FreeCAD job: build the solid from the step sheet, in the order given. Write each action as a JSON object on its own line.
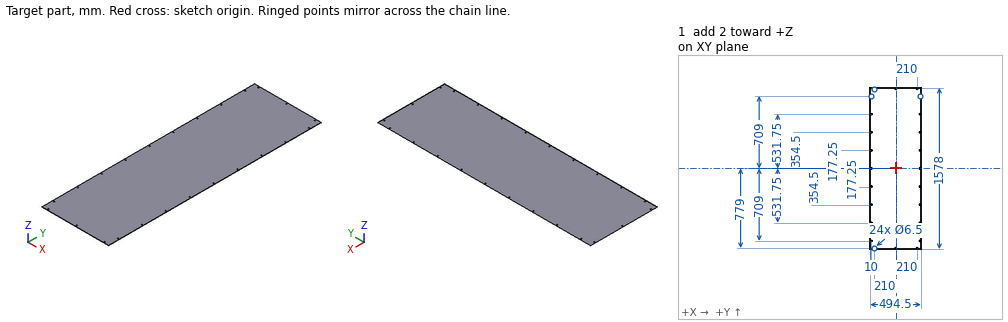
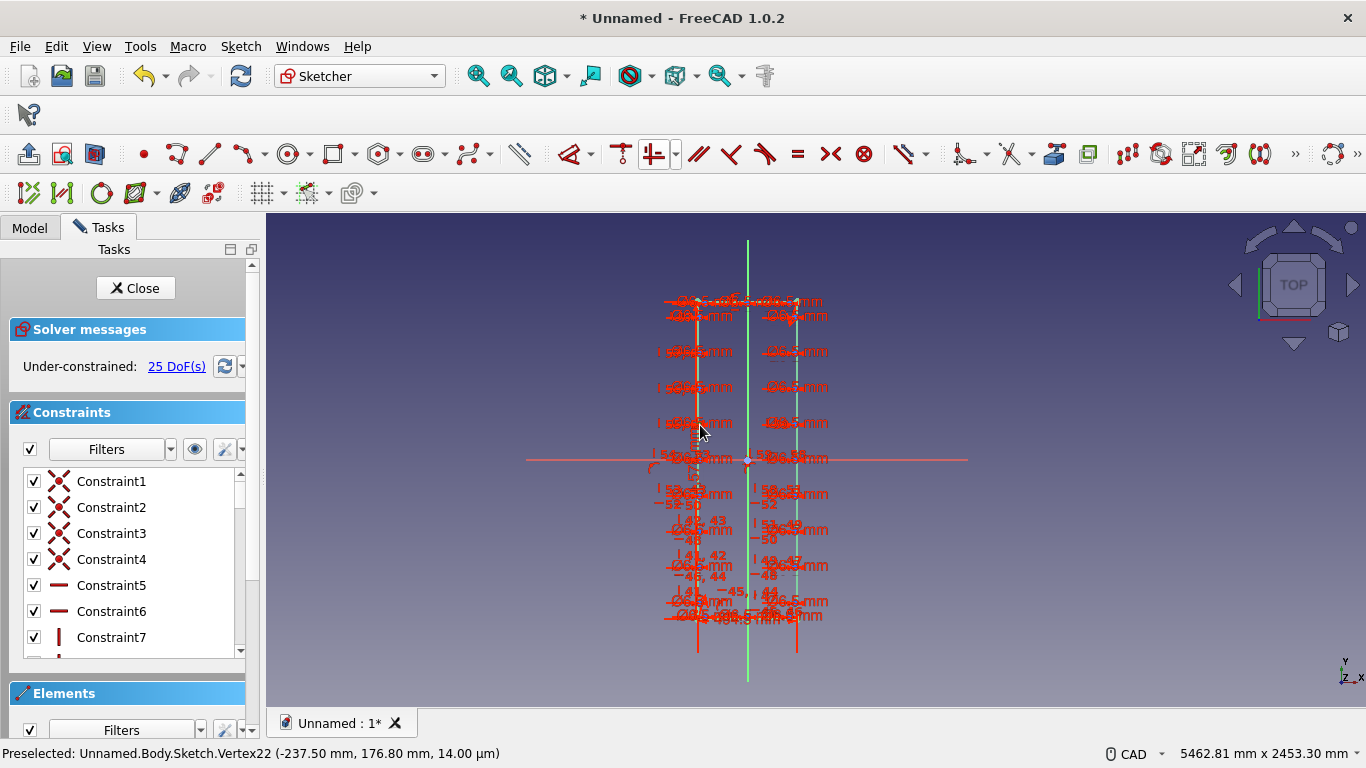
{"action": "left_click", "coordinate": [795, 425]}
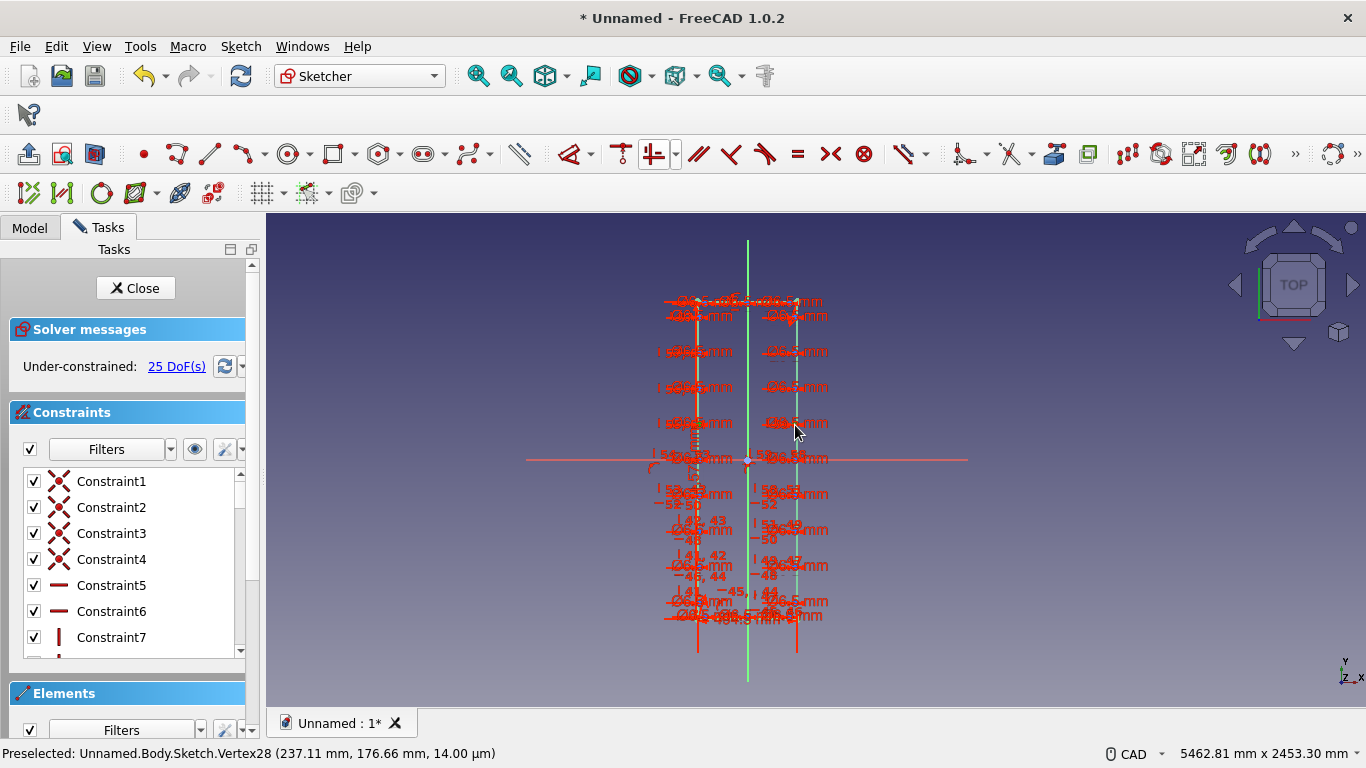
{"action": "left_click", "coordinate": [676, 154]}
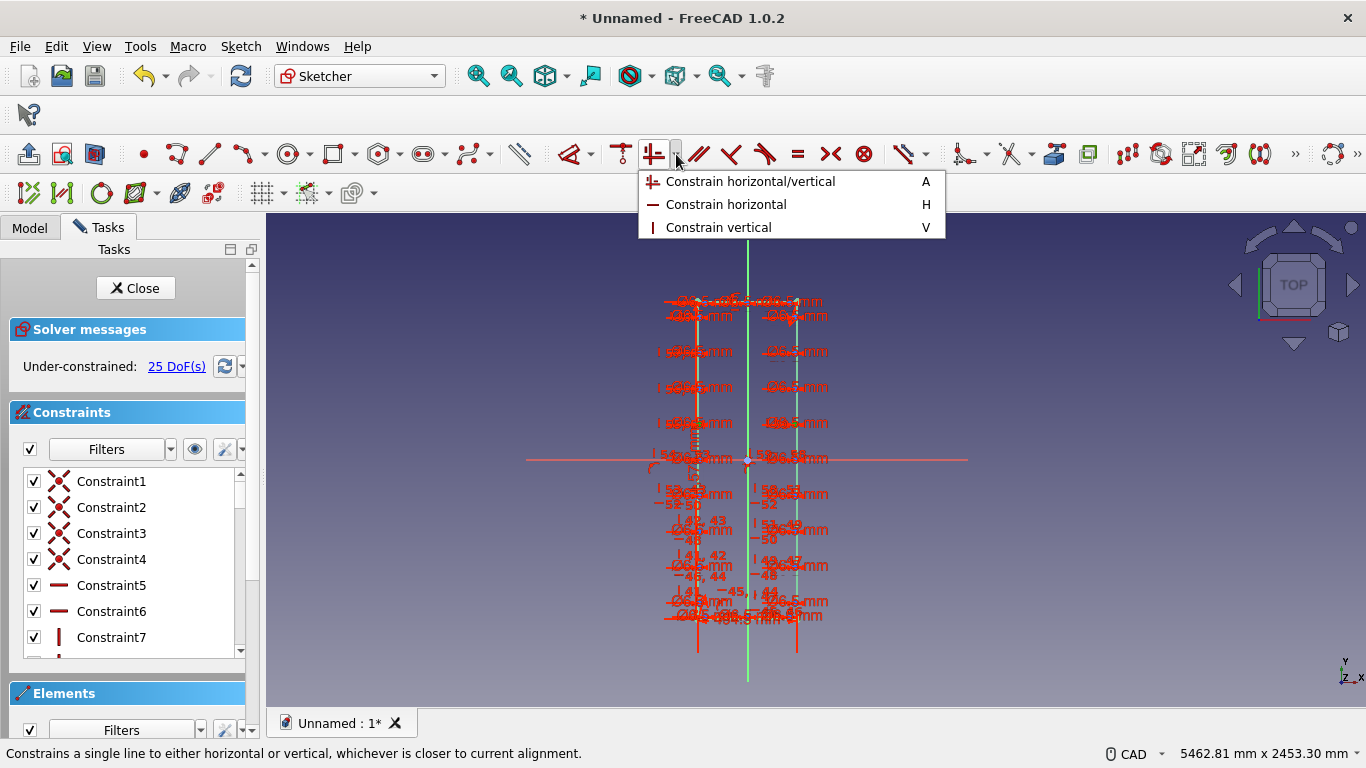
{"action": "left_click", "coordinate": [792, 204]}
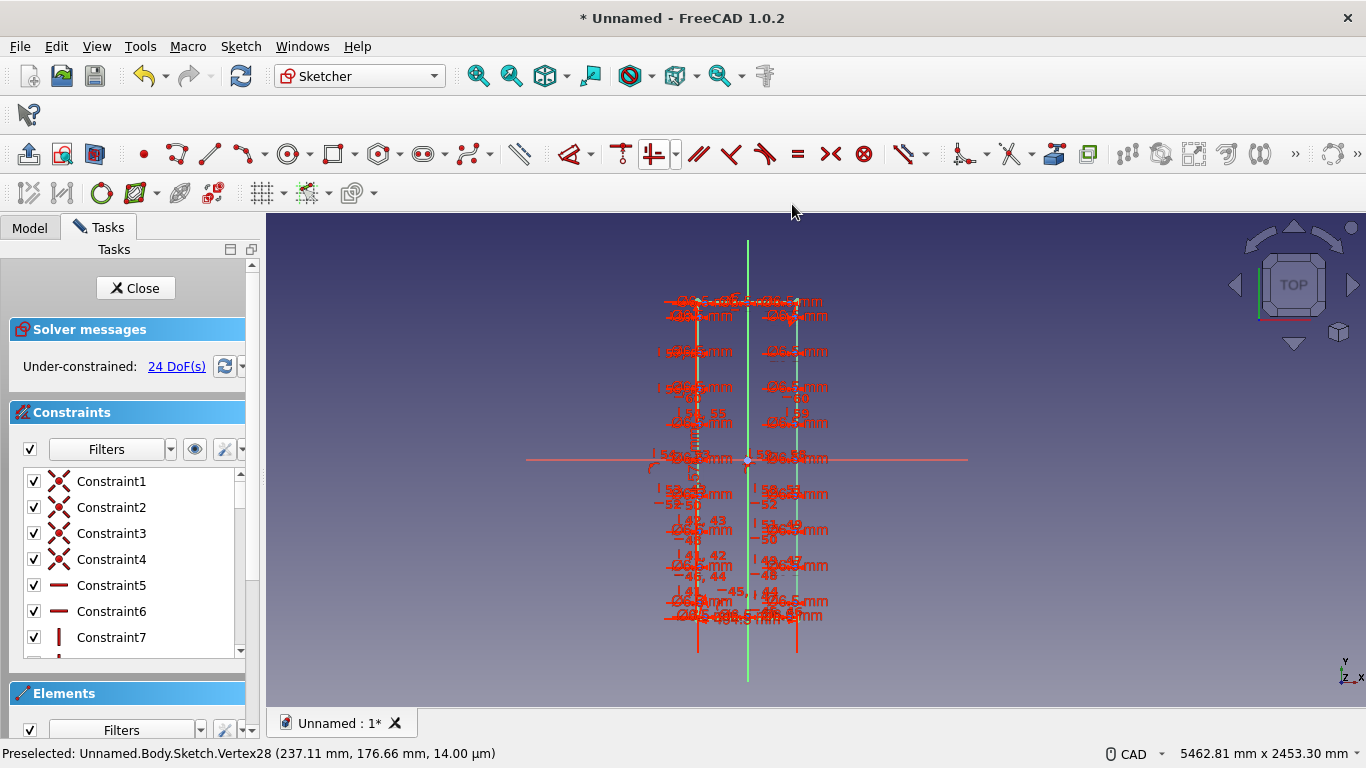
{"action": "left_click", "coordinate": [795, 425]}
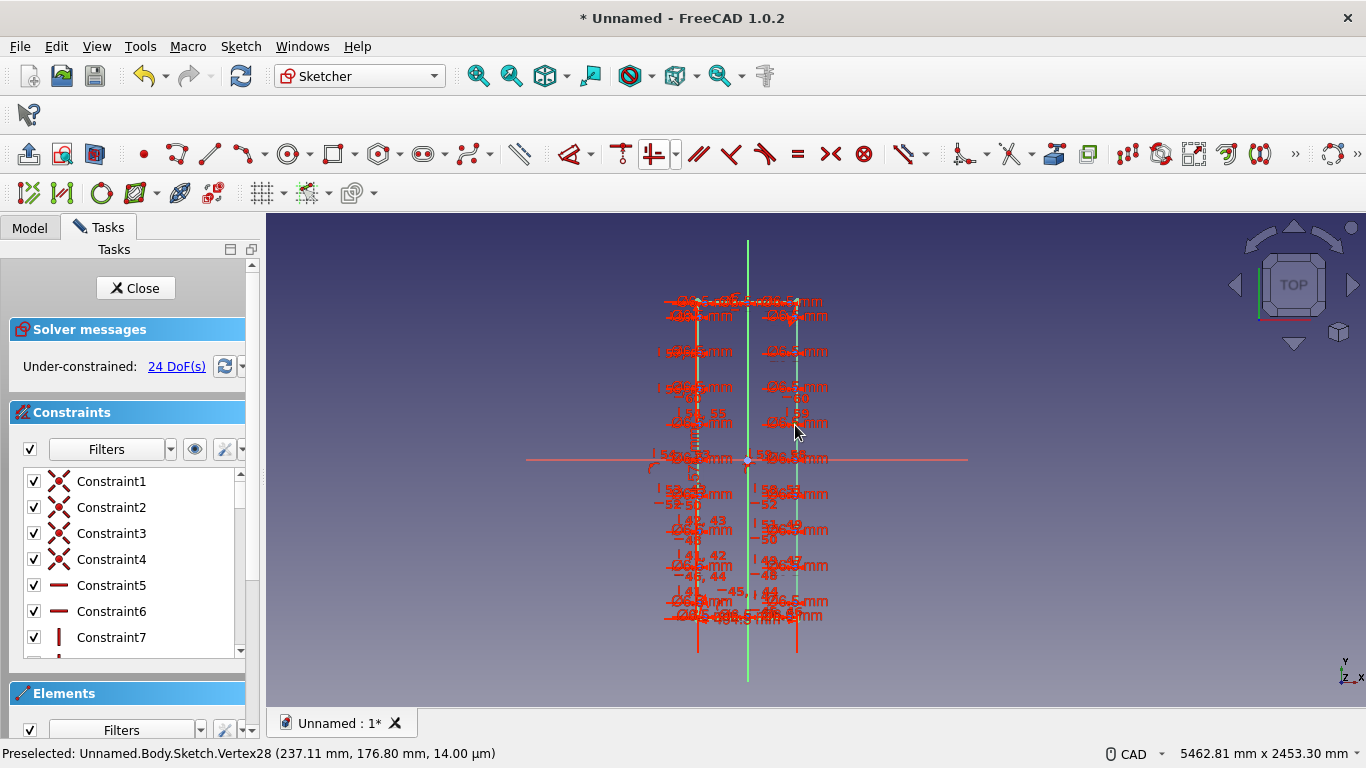
{"action": "left_click", "coordinate": [795, 389]}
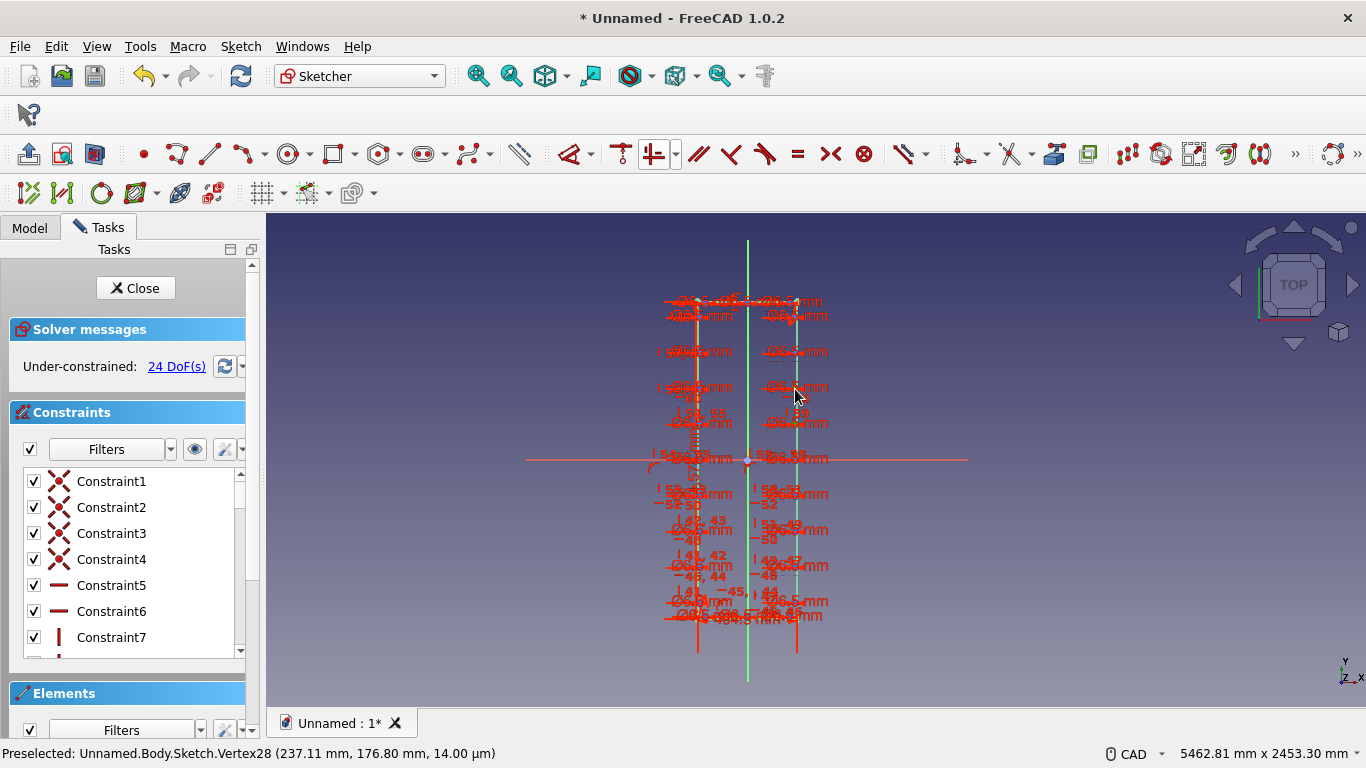
{"action": "key", "text": "v"}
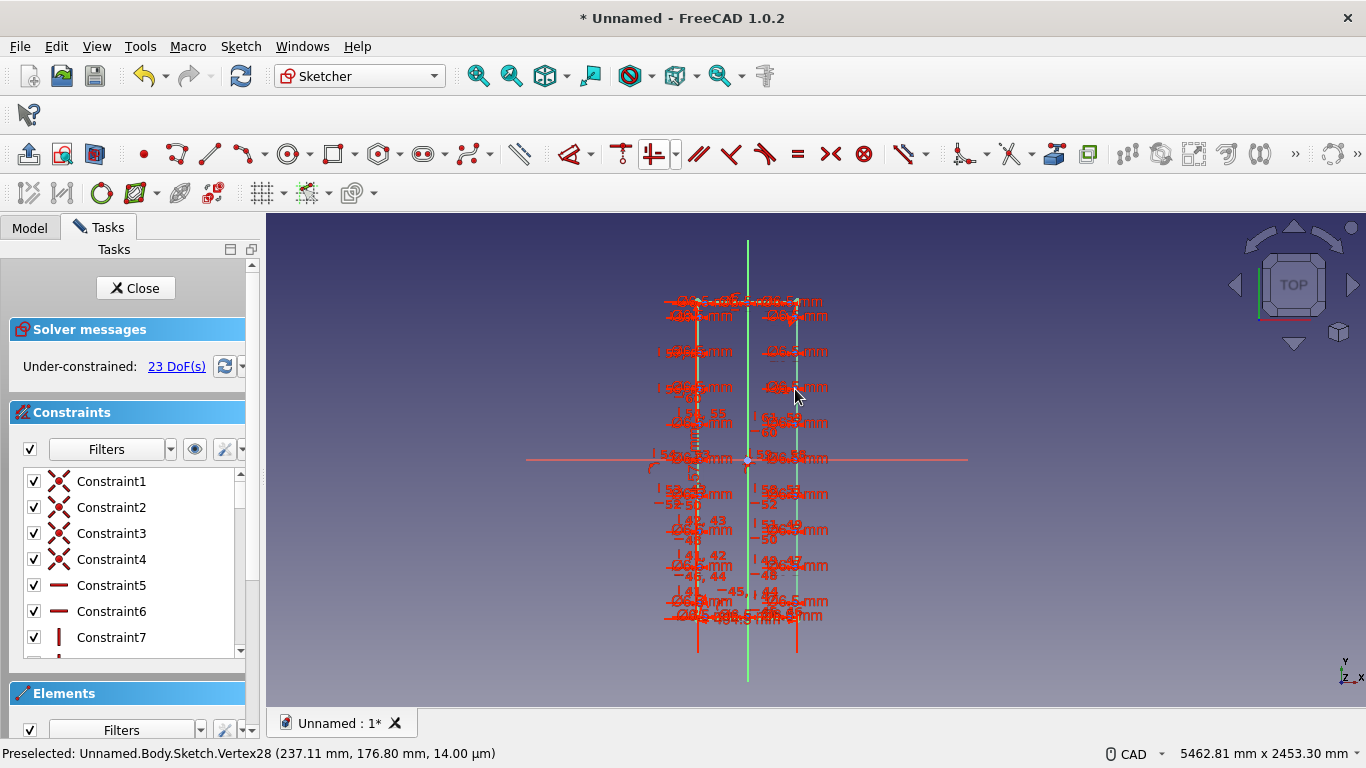
{"action": "left_click", "coordinate": [700, 389]}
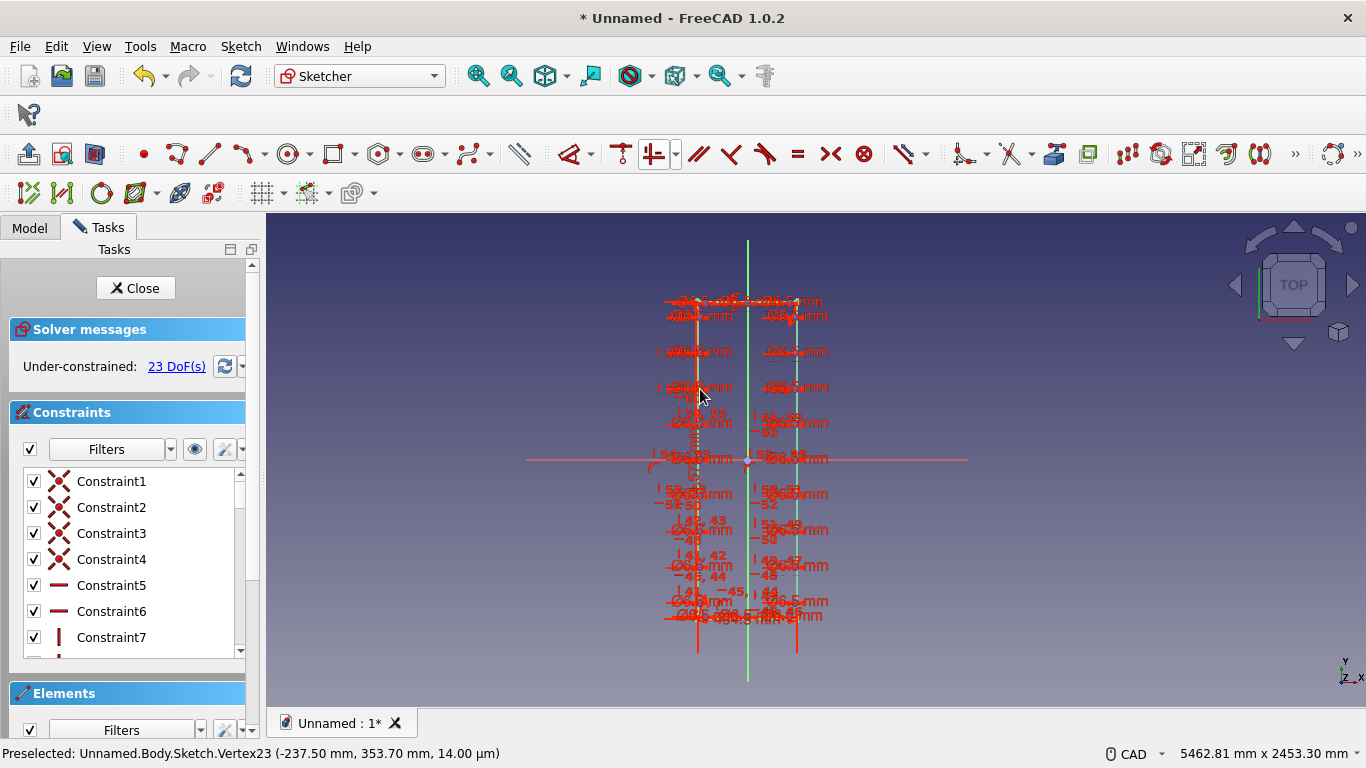
{"action": "left_click", "coordinate": [795, 389]}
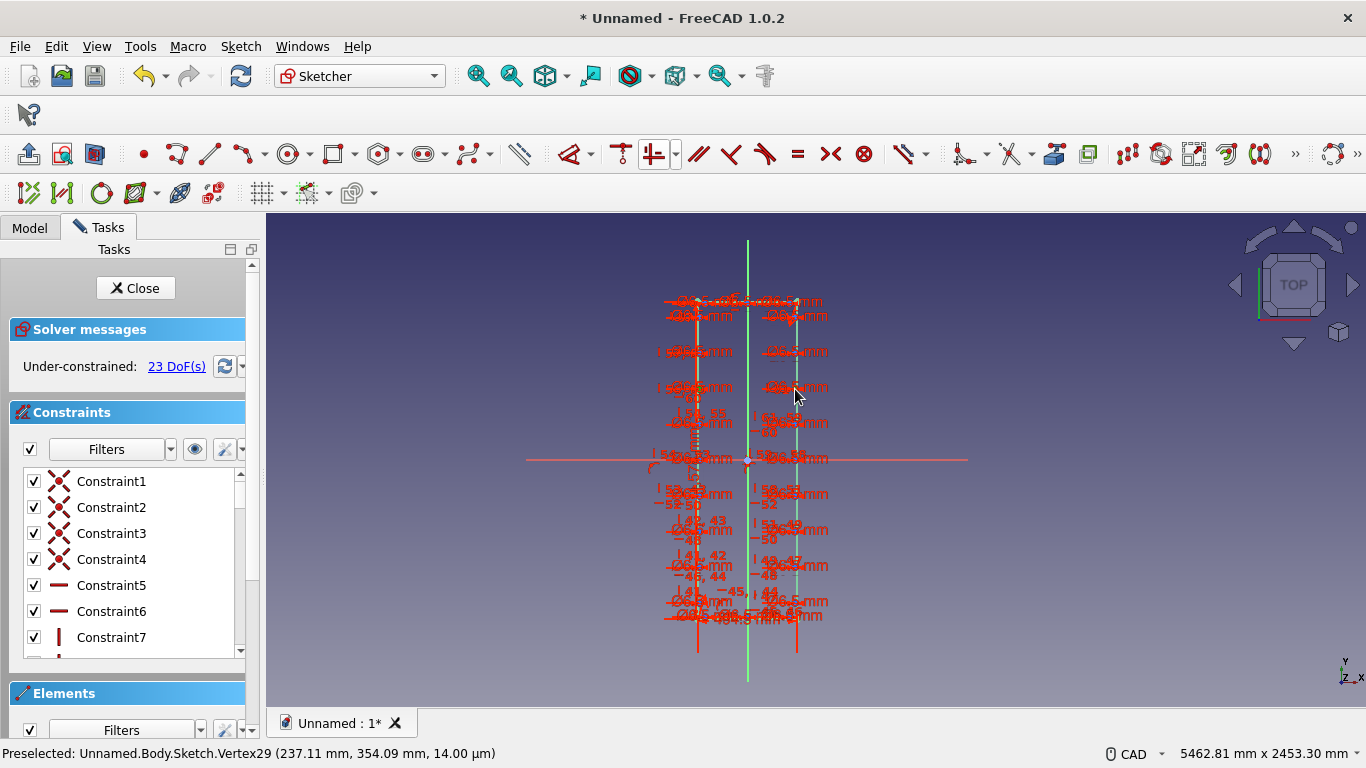
{"action": "key", "text": "h"}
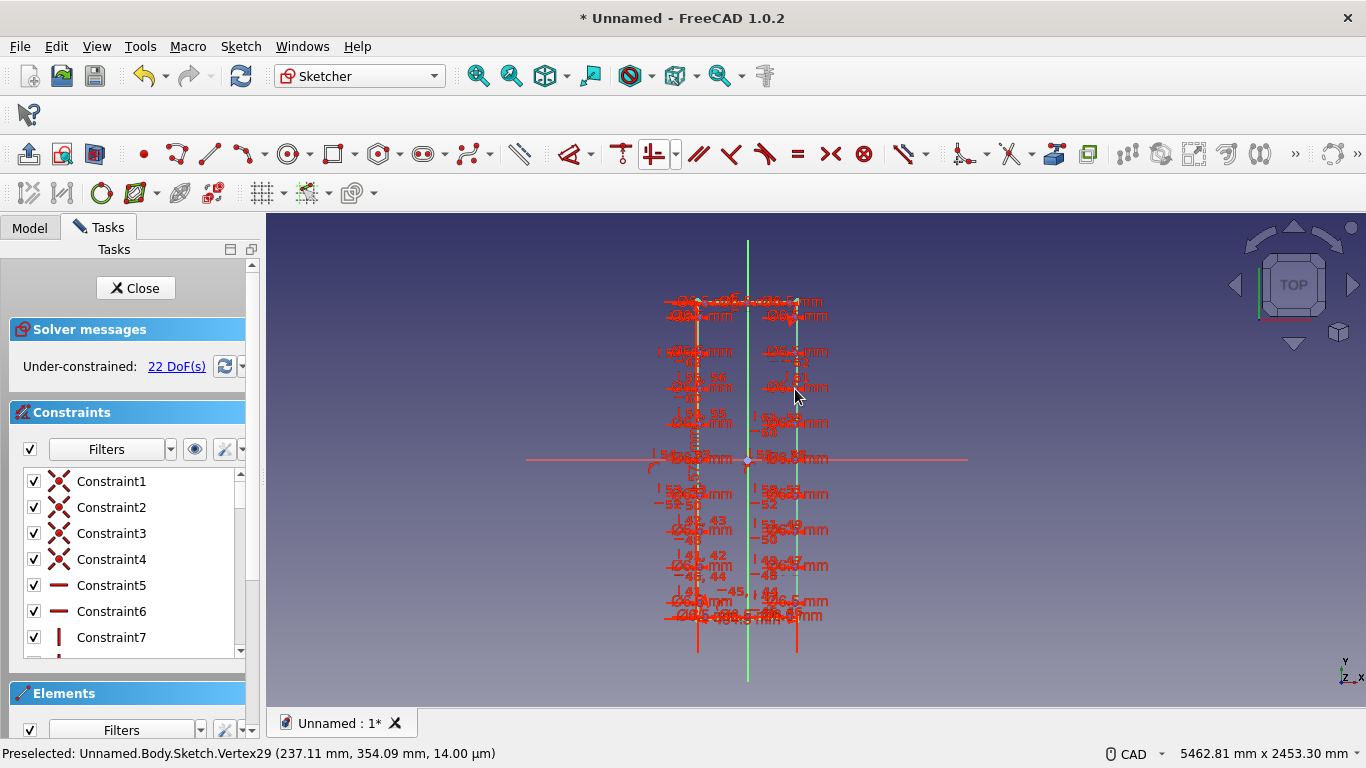
{"action": "scroll", "coordinate": [705, 304], "scroll_direction": "up", "scroll_amount": 3}